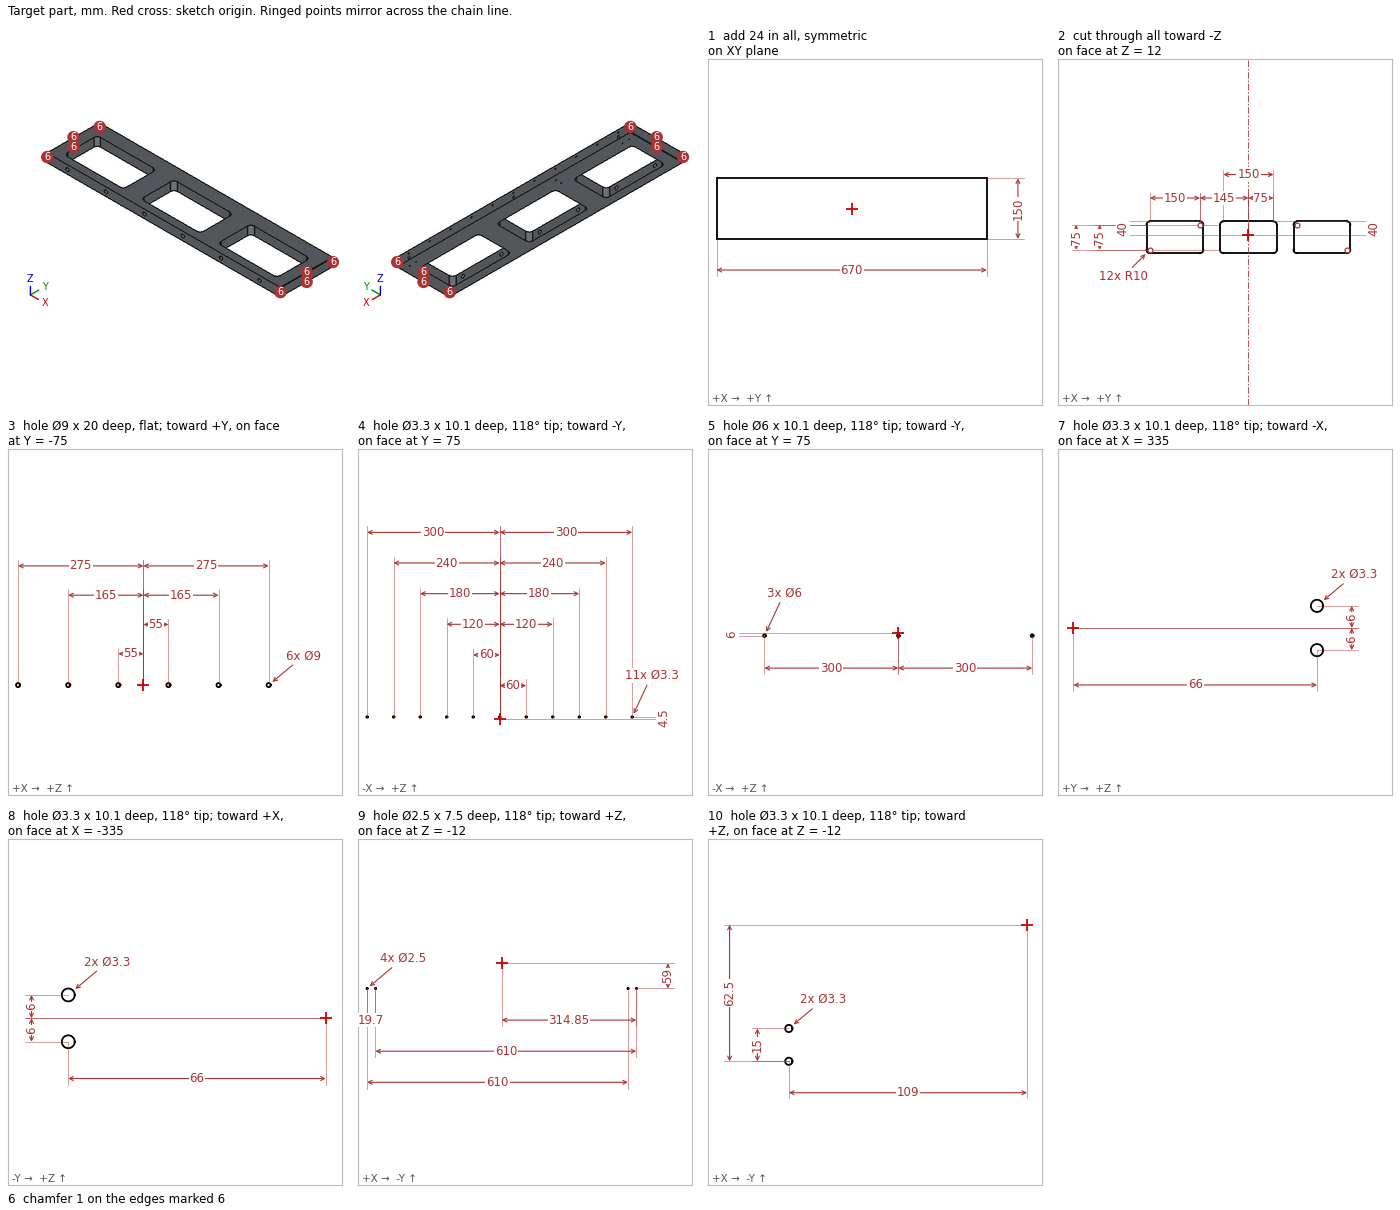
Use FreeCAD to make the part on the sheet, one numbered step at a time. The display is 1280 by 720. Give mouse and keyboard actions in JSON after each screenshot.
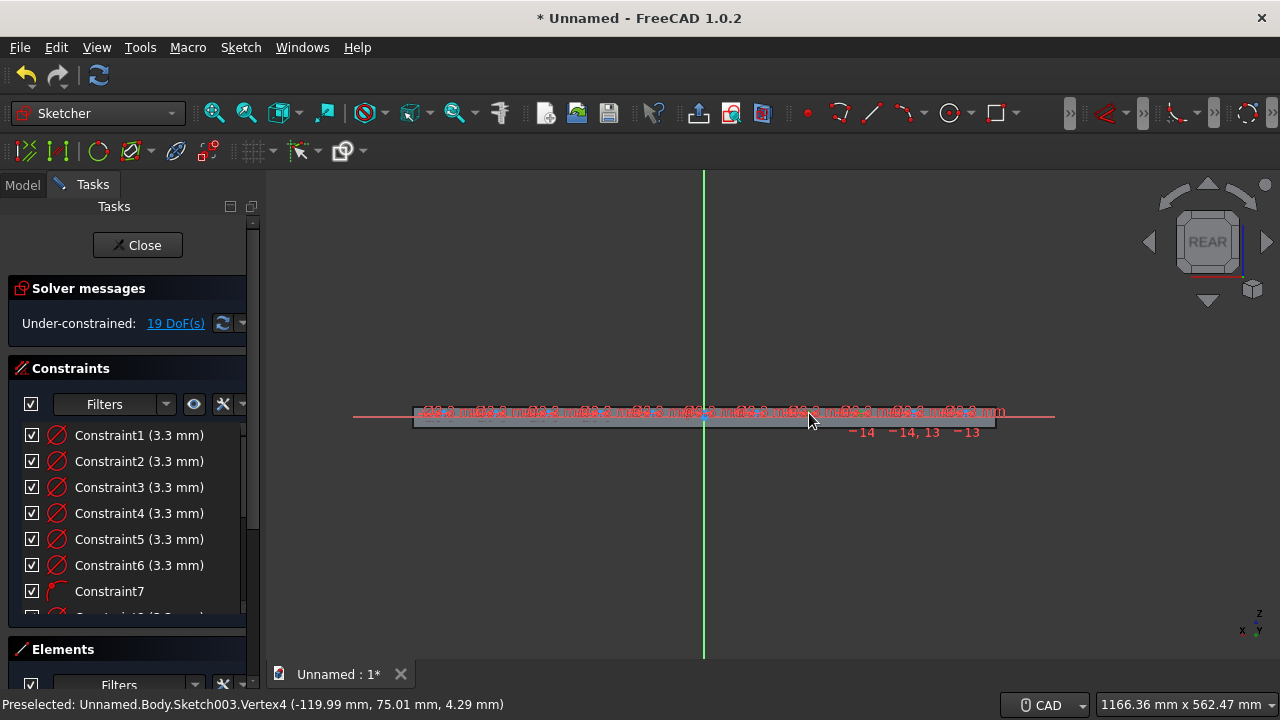
{"action": "key", "text": "h"}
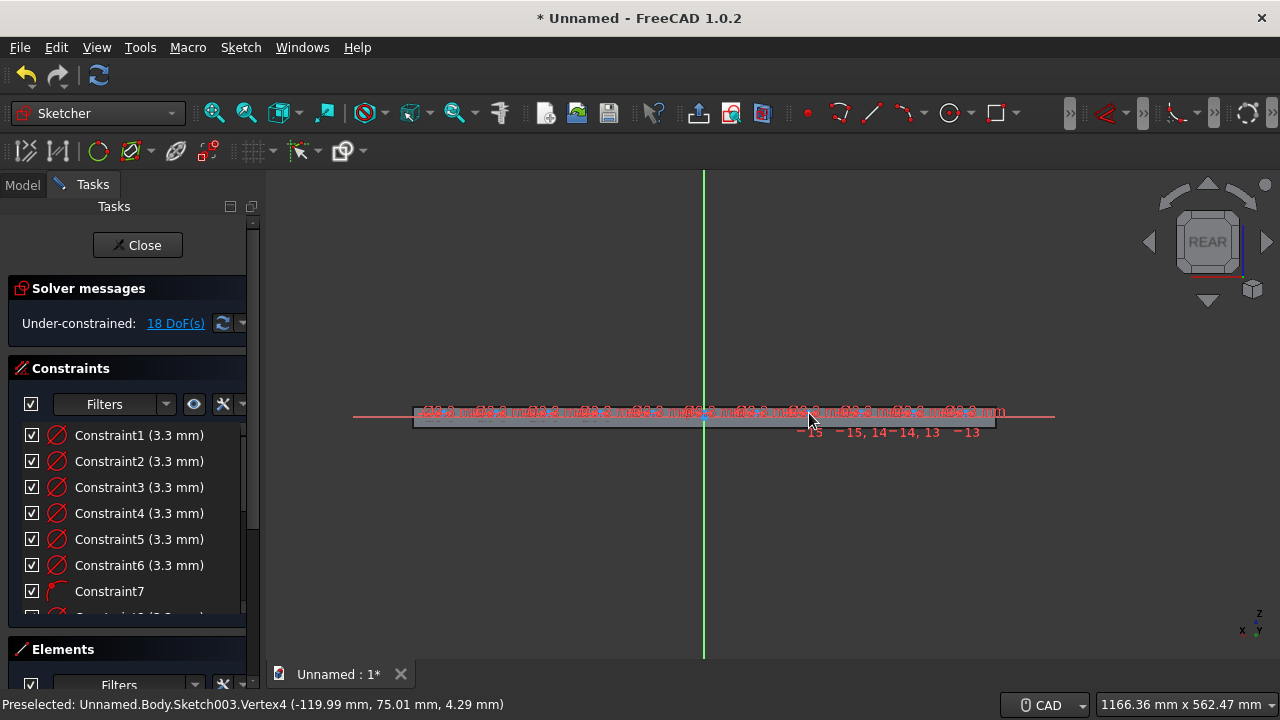
{"action": "left_click", "coordinate": [809, 413]}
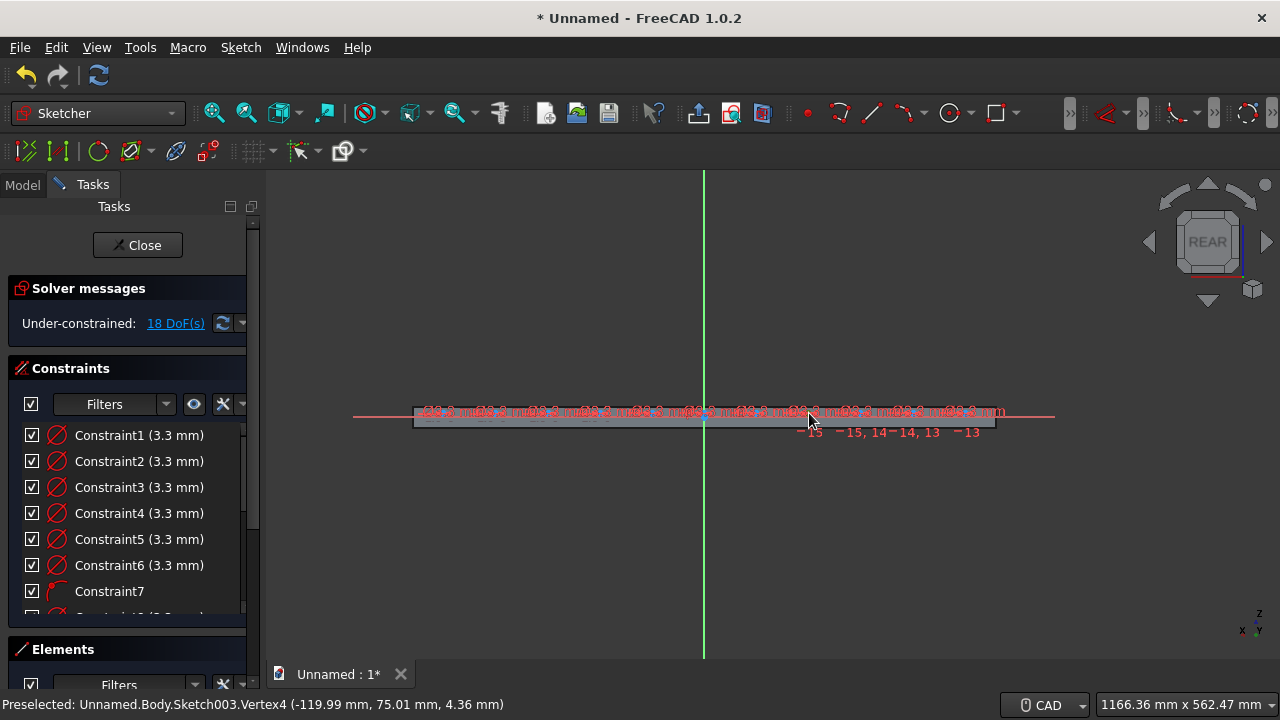
{"action": "left_click", "coordinate": [757, 413]}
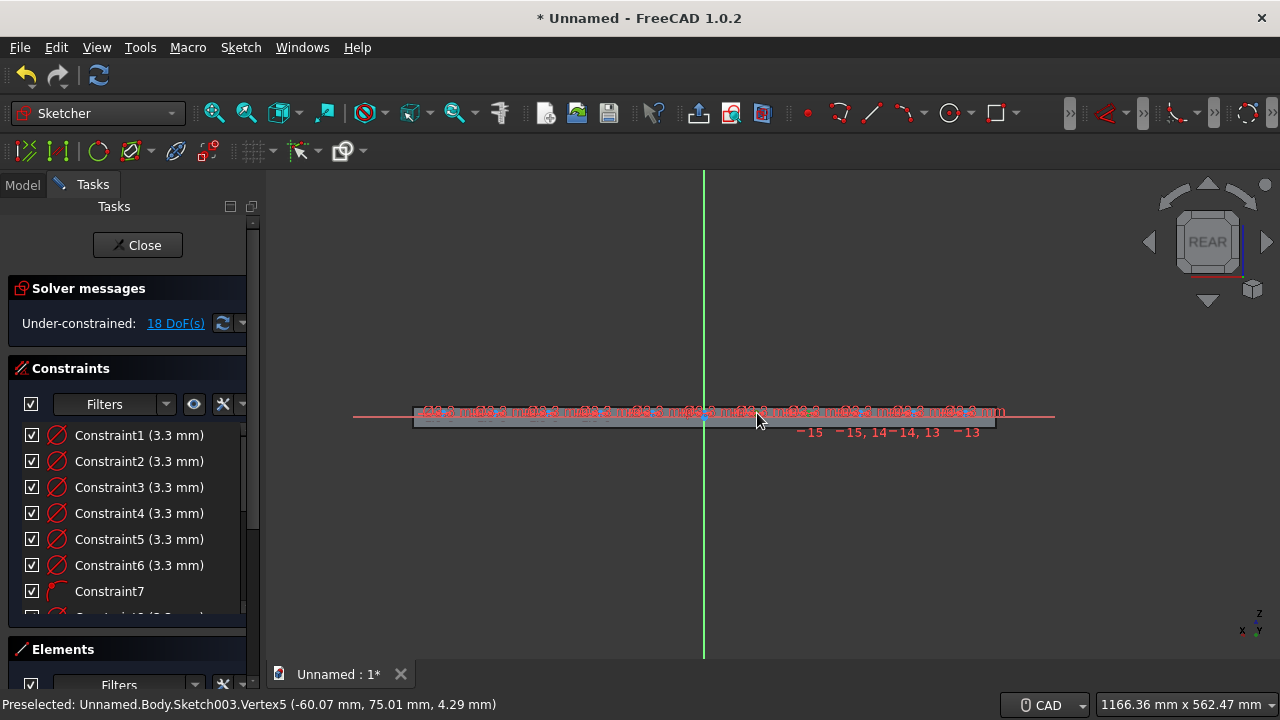
{"action": "key", "text": "h"}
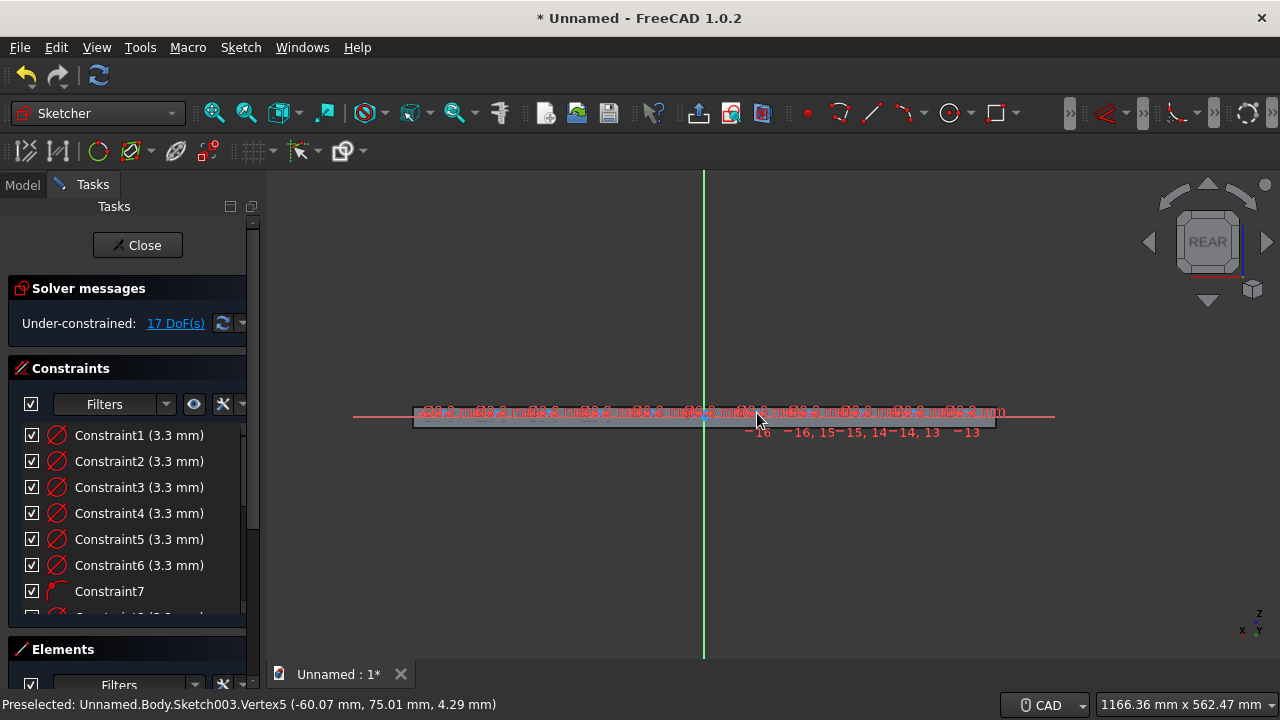
{"action": "left_click", "coordinate": [757, 413]}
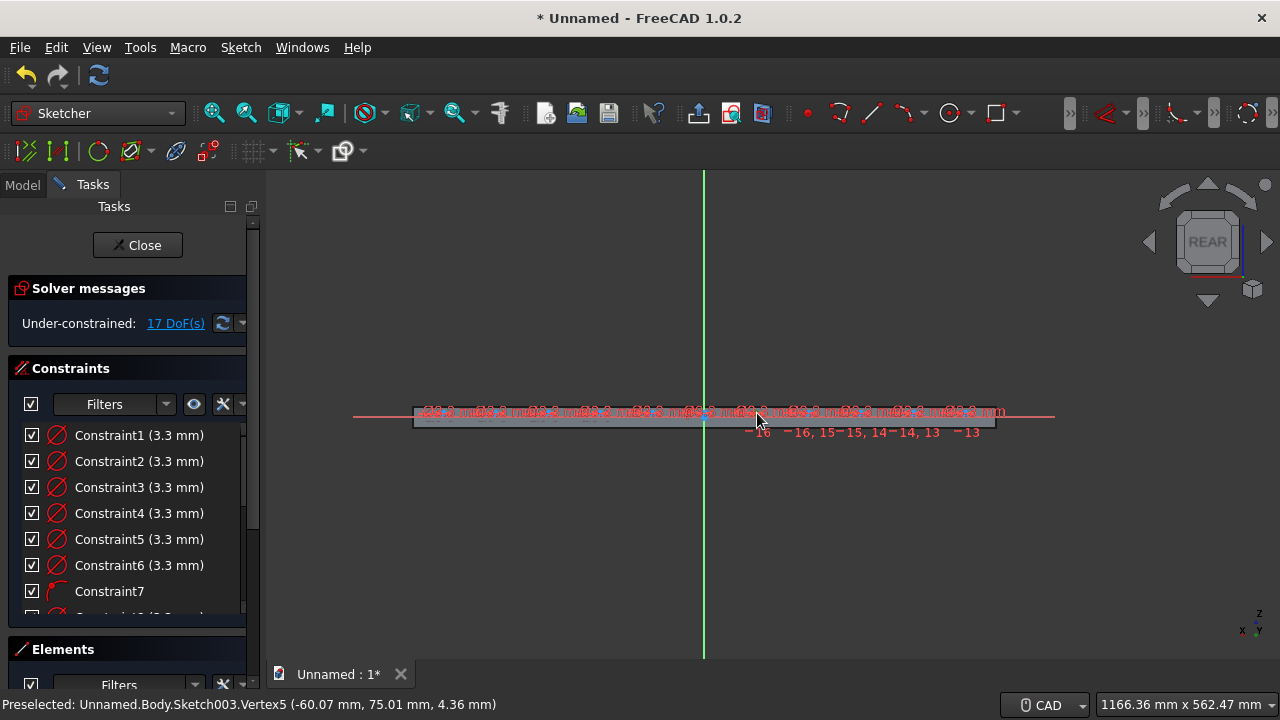
{"action": "scroll", "coordinate": [704, 413], "scroll_direction": "up", "scroll_amount": 6}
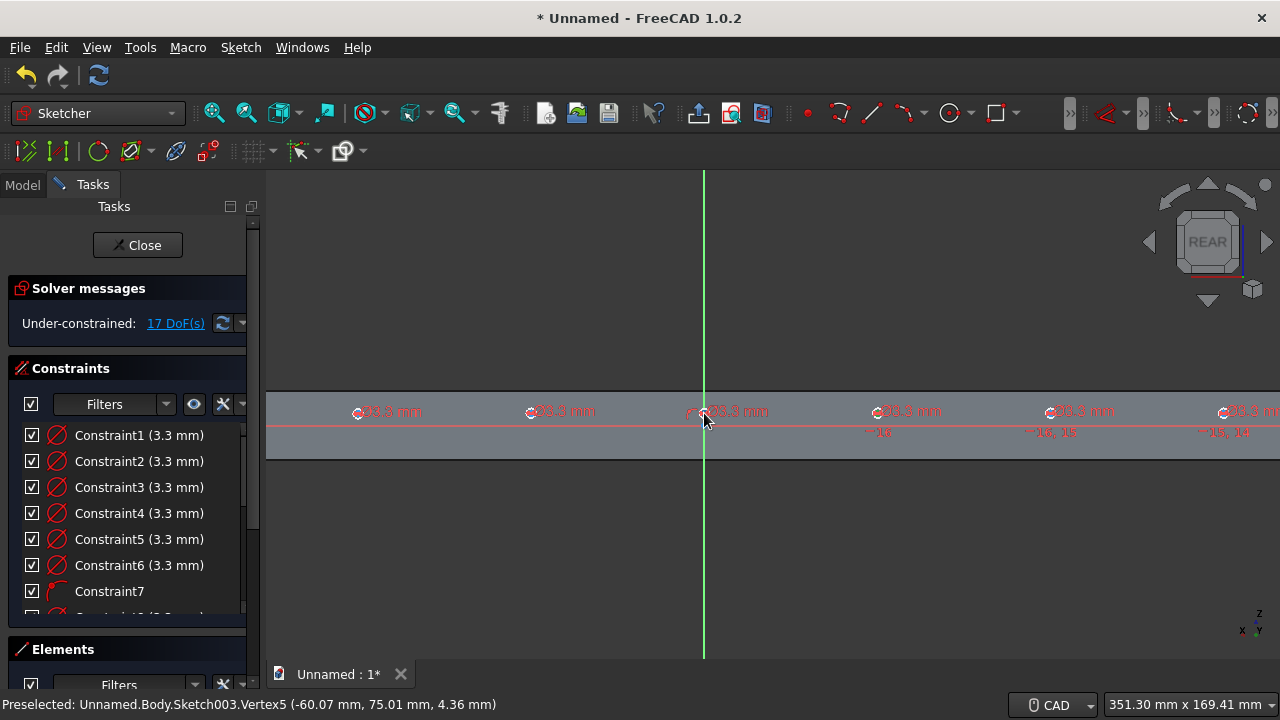
{"action": "left_click", "coordinate": [704, 413]}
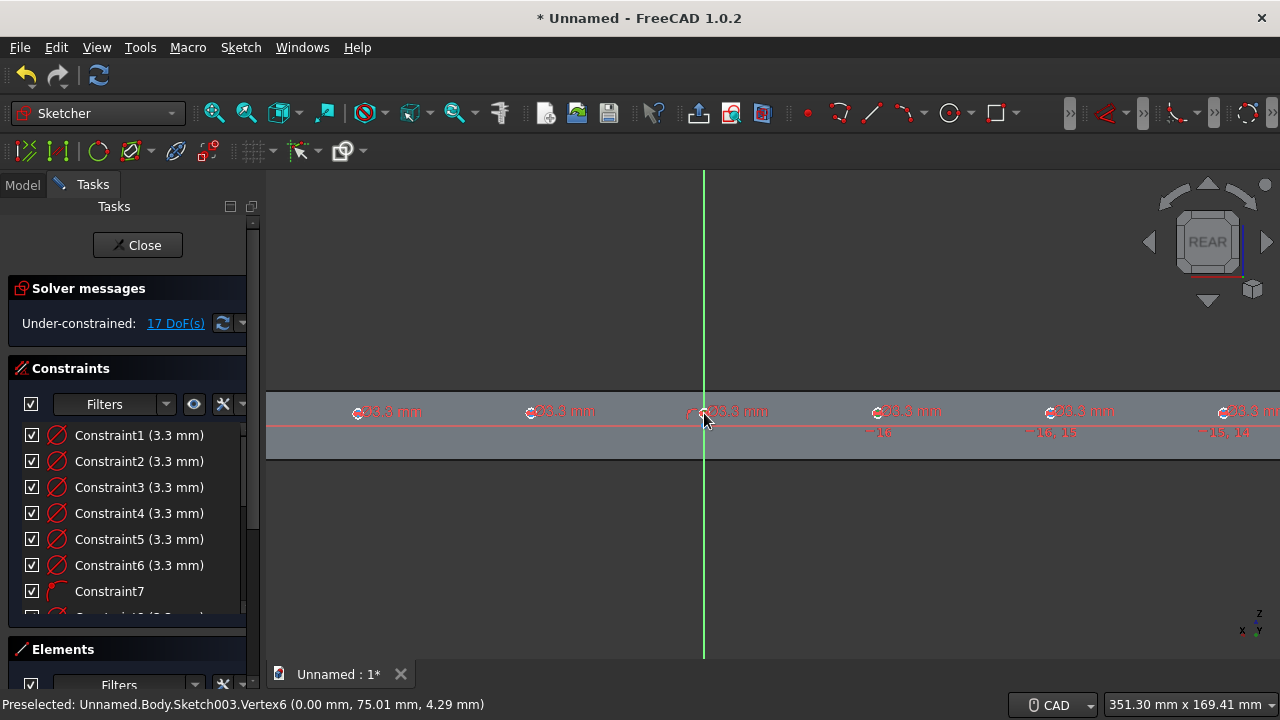
{"action": "key", "text": "h"}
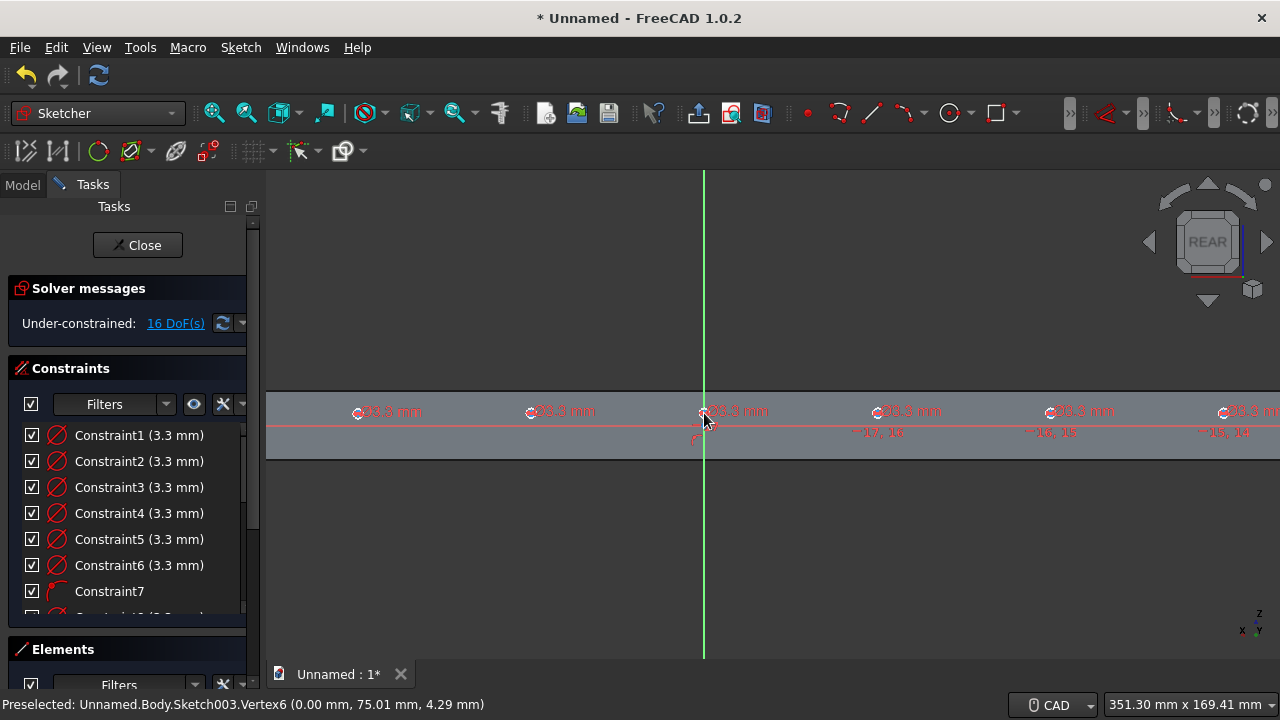
{"action": "left_click", "coordinate": [704, 413]}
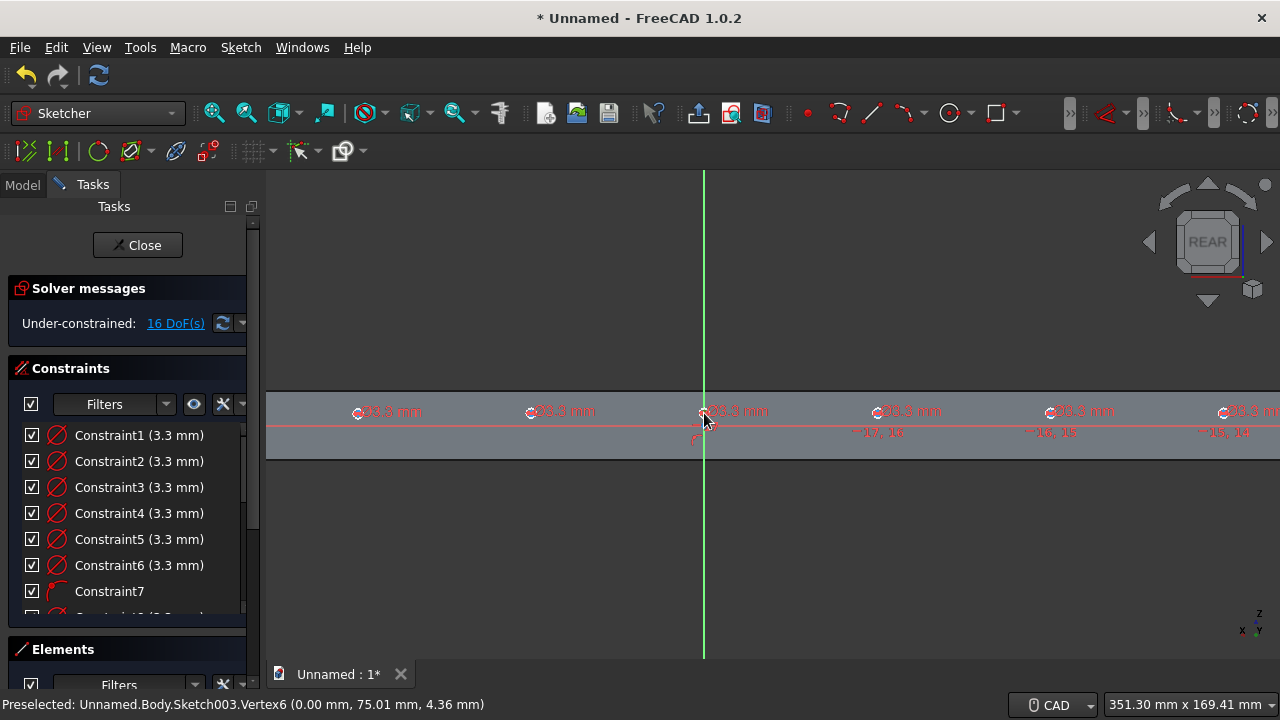
{"action": "scroll", "coordinate": [705, 413], "scroll_direction": "down", "scroll_amount": 6}